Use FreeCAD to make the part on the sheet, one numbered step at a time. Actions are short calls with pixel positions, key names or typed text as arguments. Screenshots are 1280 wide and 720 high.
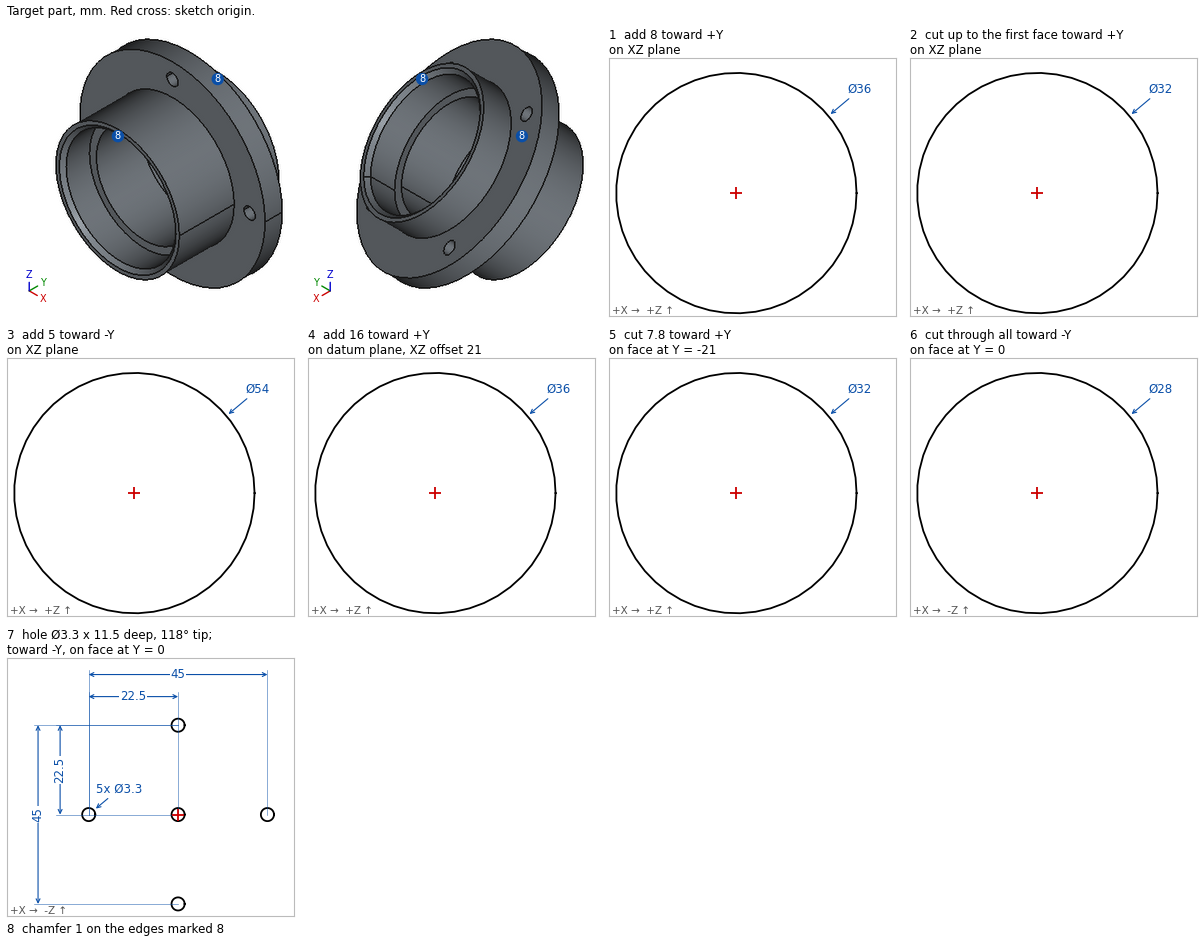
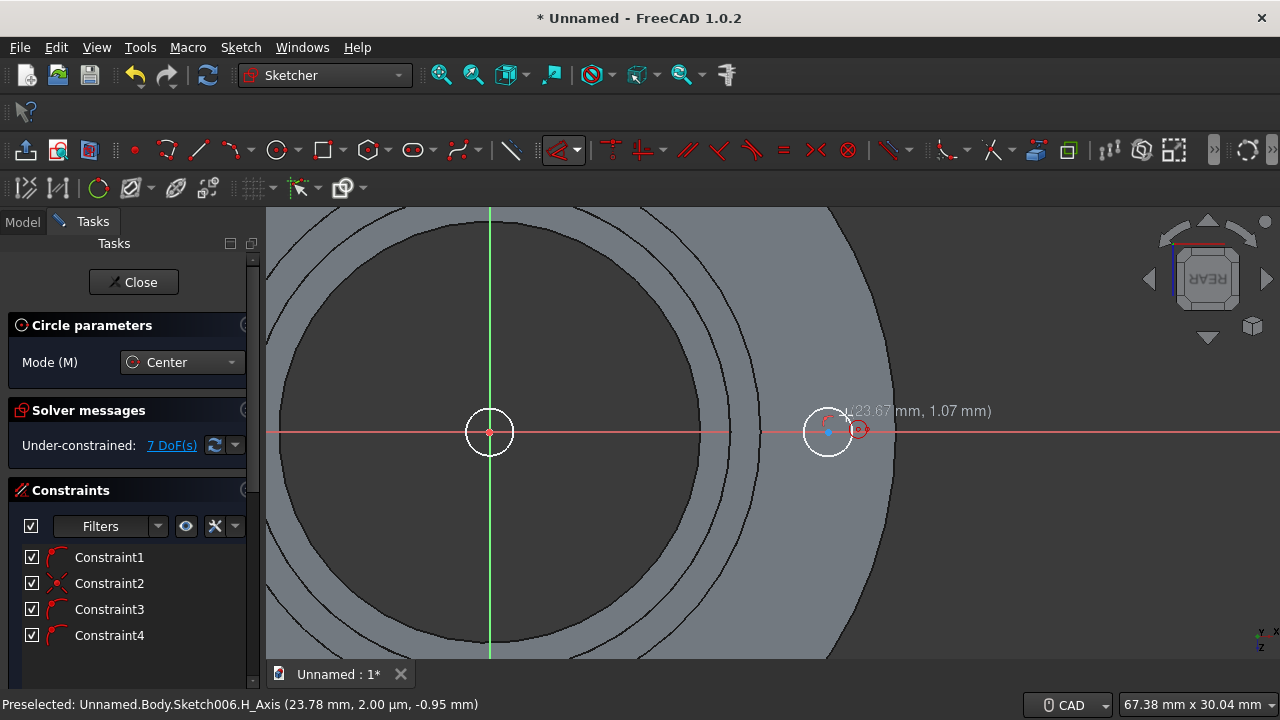
scroll(829, 434, down, 5)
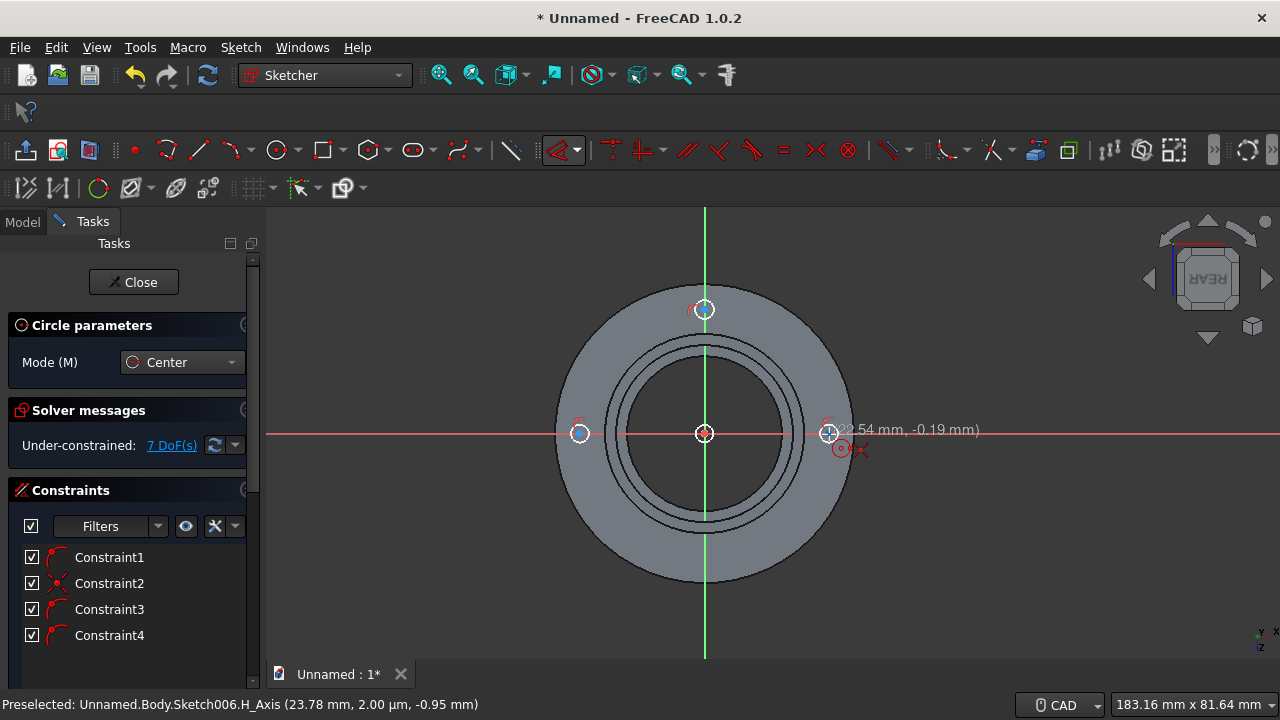
scroll(705, 558, up, 5)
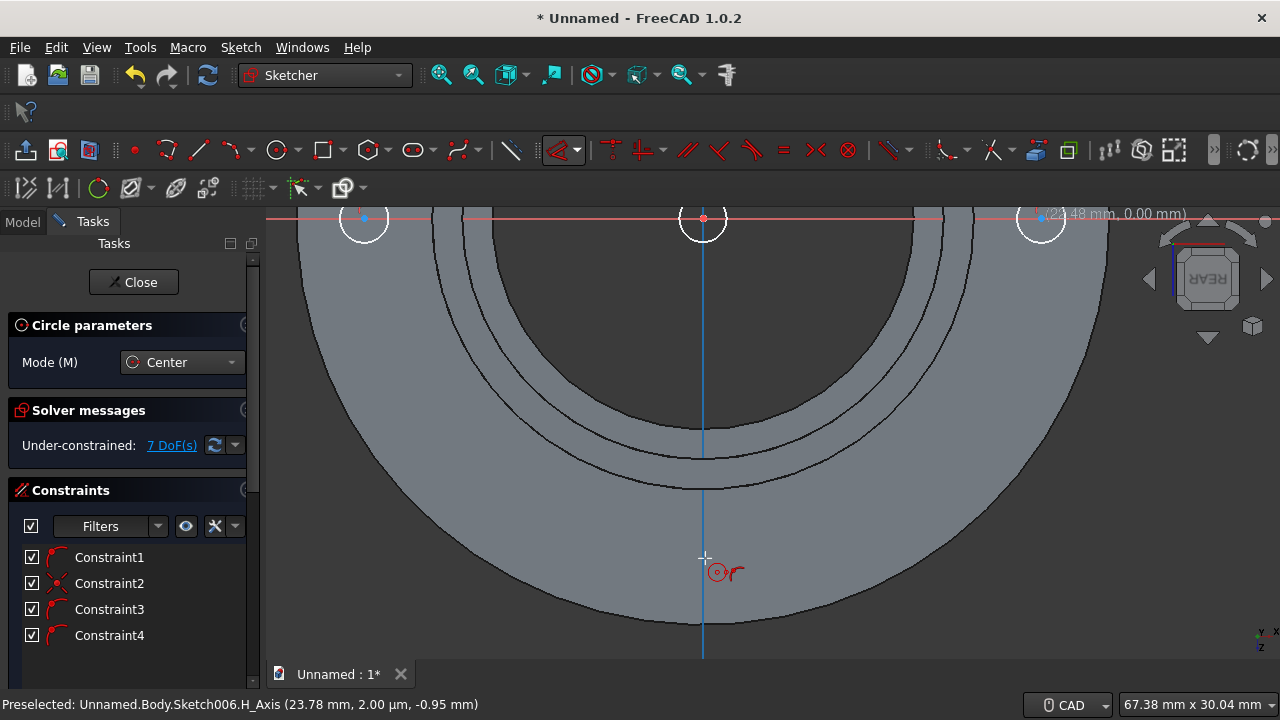
click(703, 557)
click(721, 540)
key(Escape)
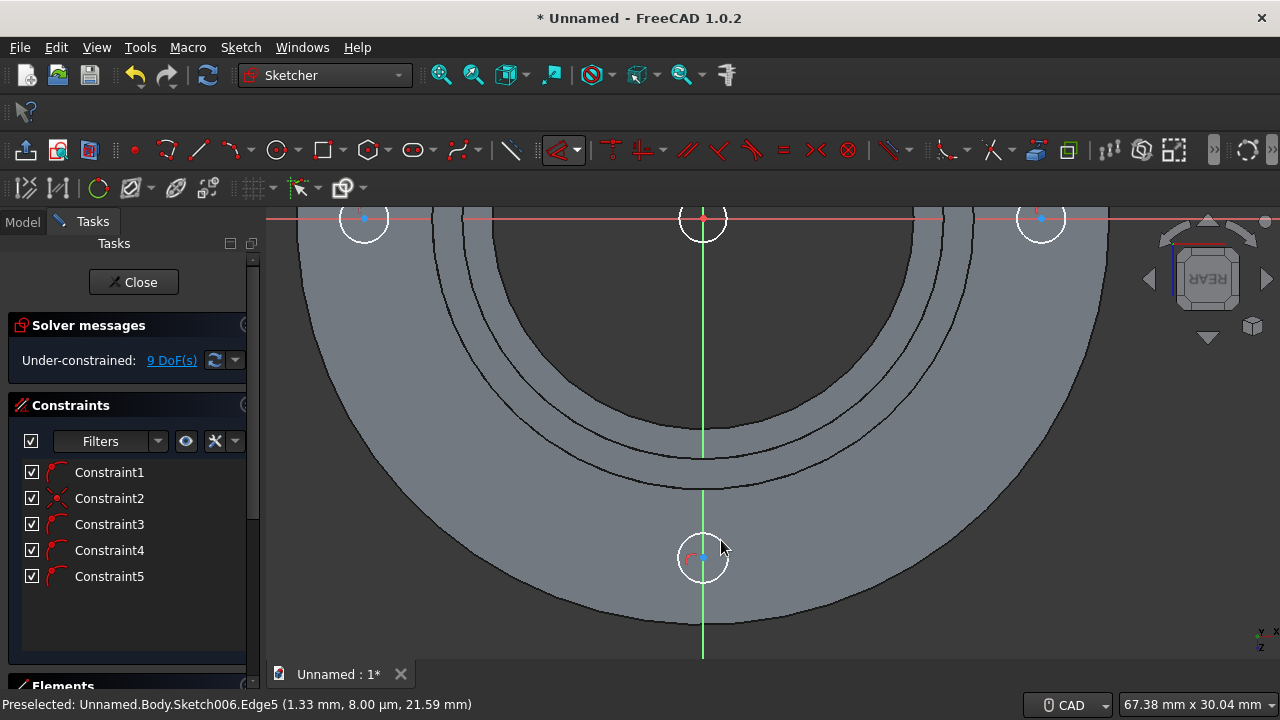
click(347, 236)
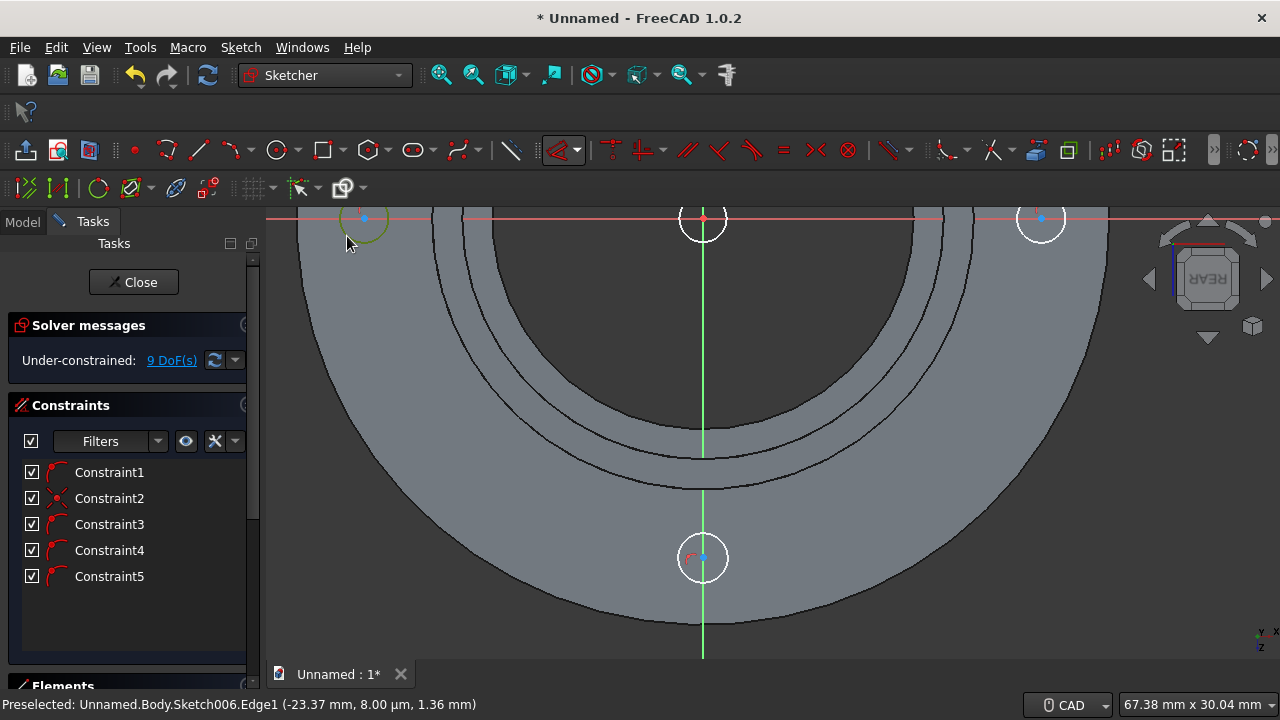
click(686, 235)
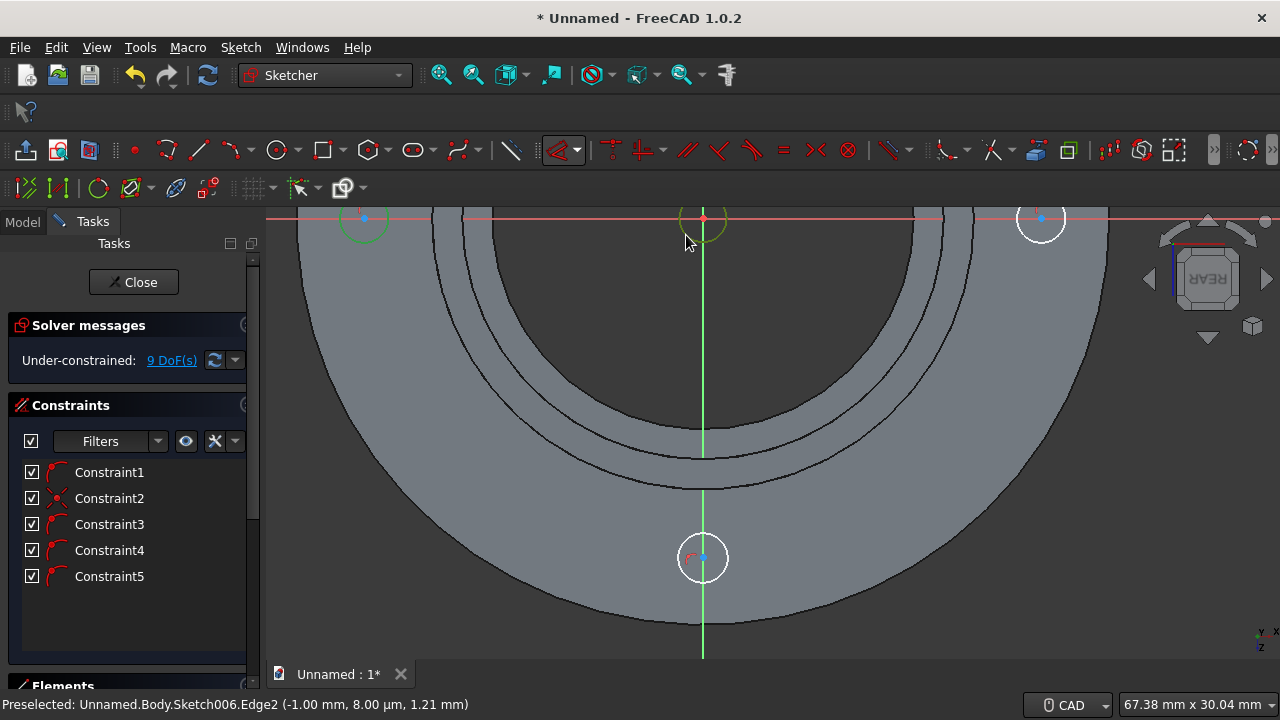
scroll(705, 558, down, 5)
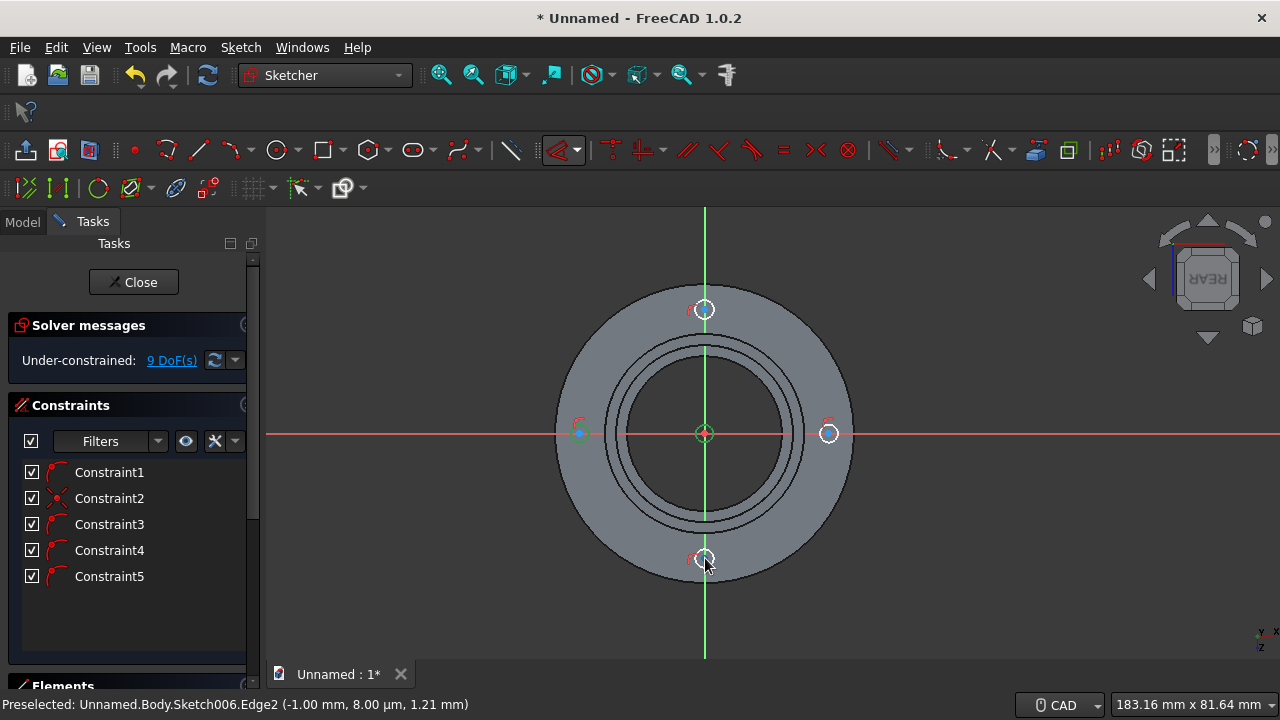
scroll(711, 303, up, 4)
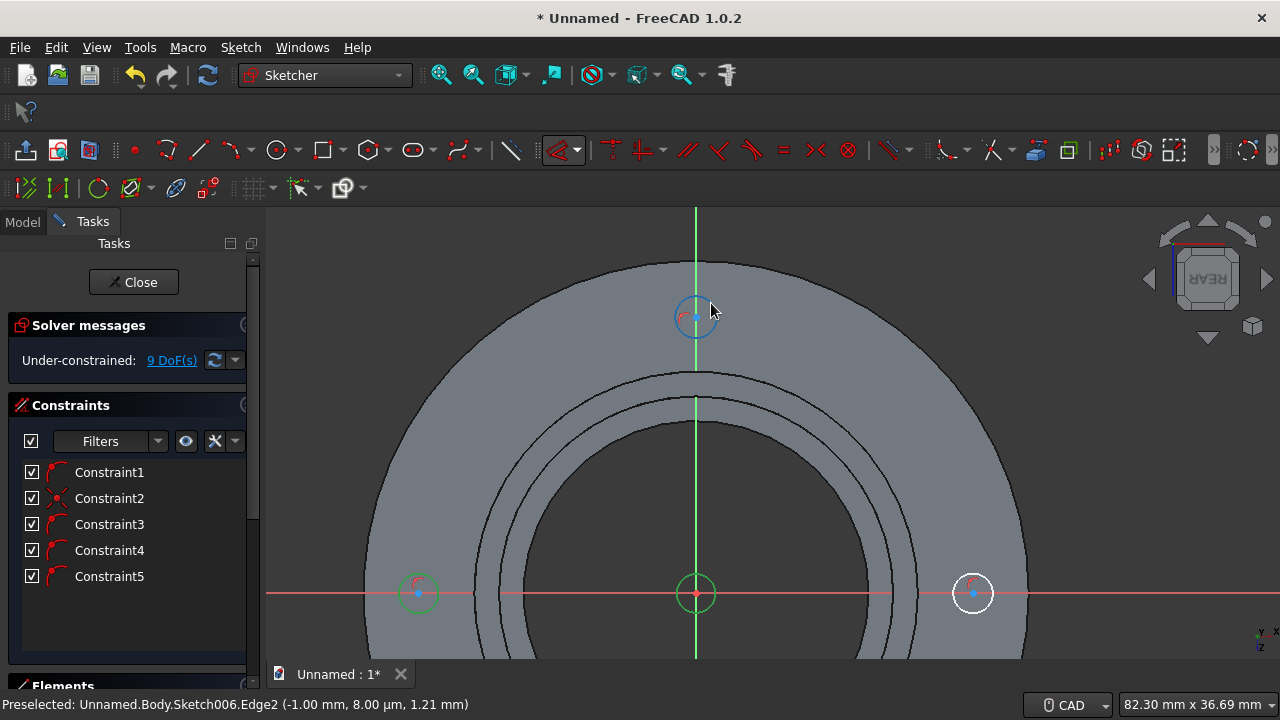
click(711, 302)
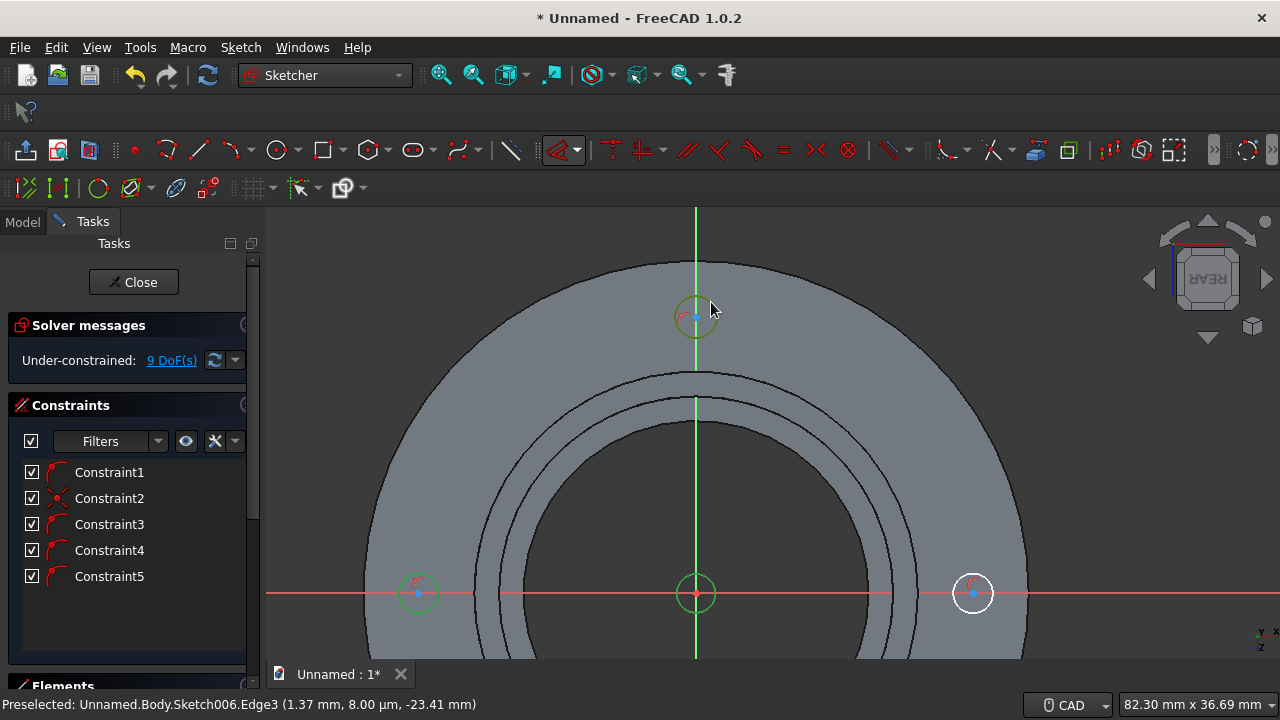
click(987, 579)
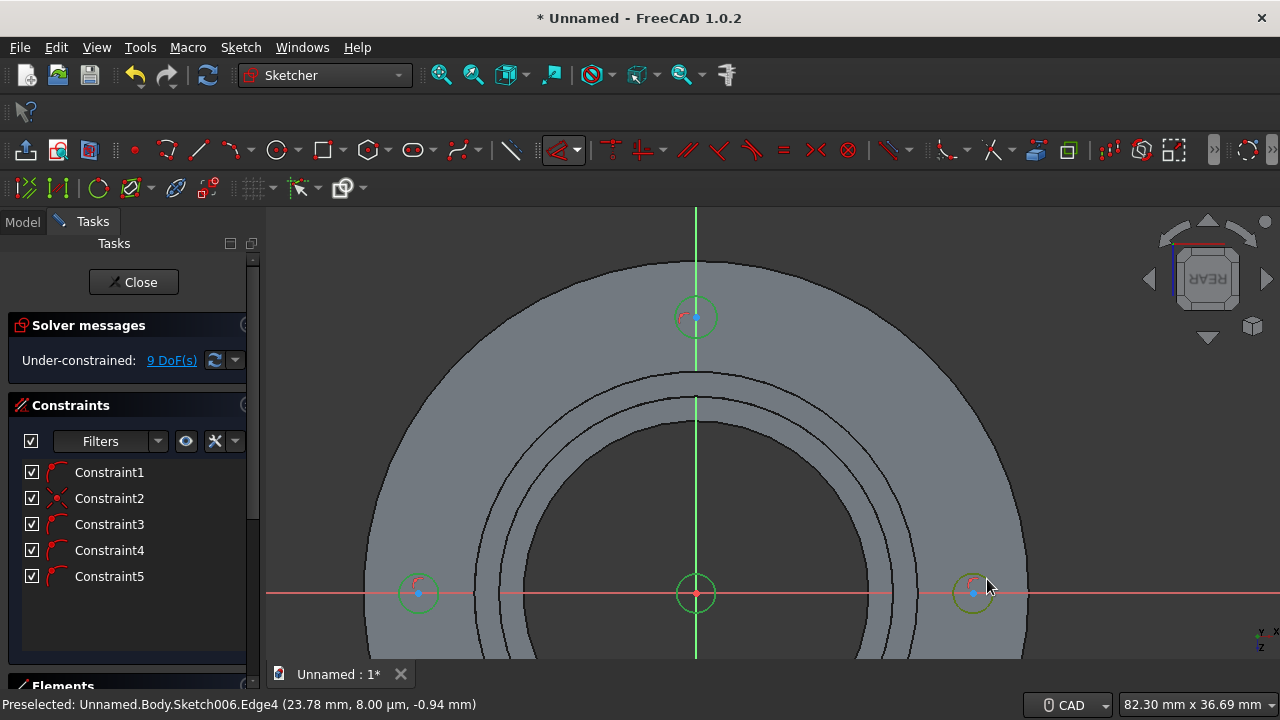
scroll(711, 302, down, 4)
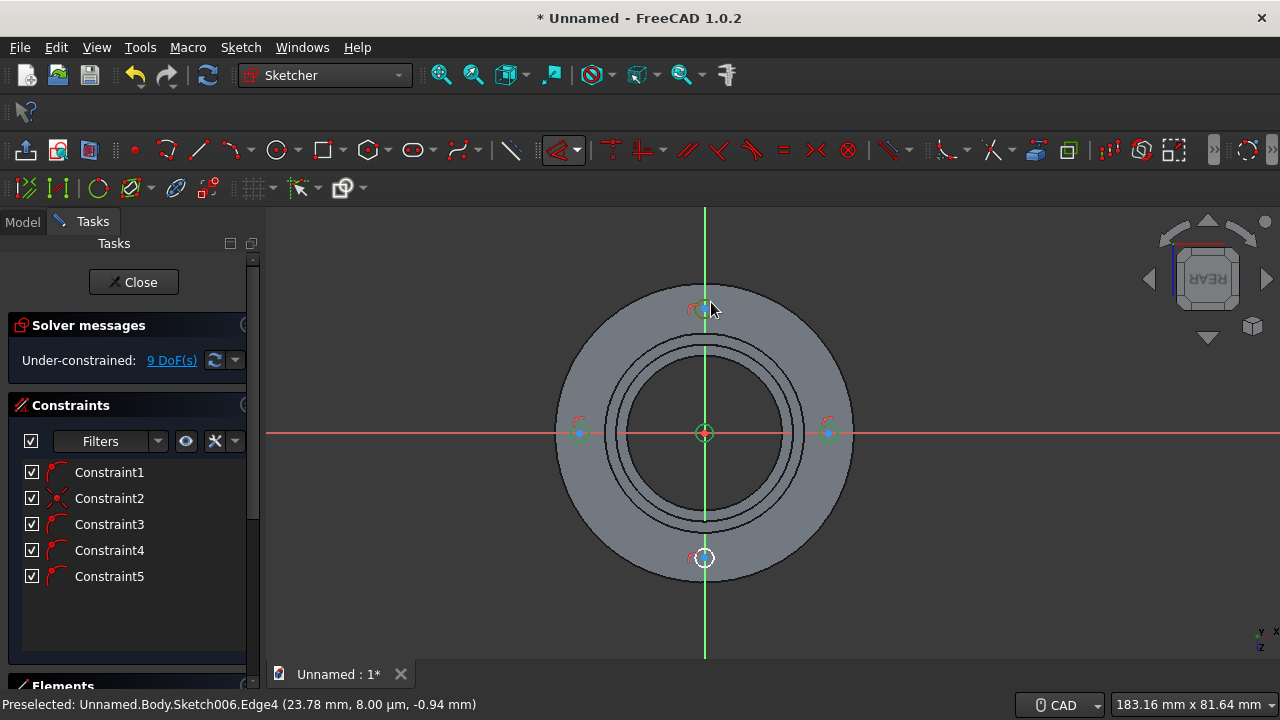
scroll(711, 551, up, 4)